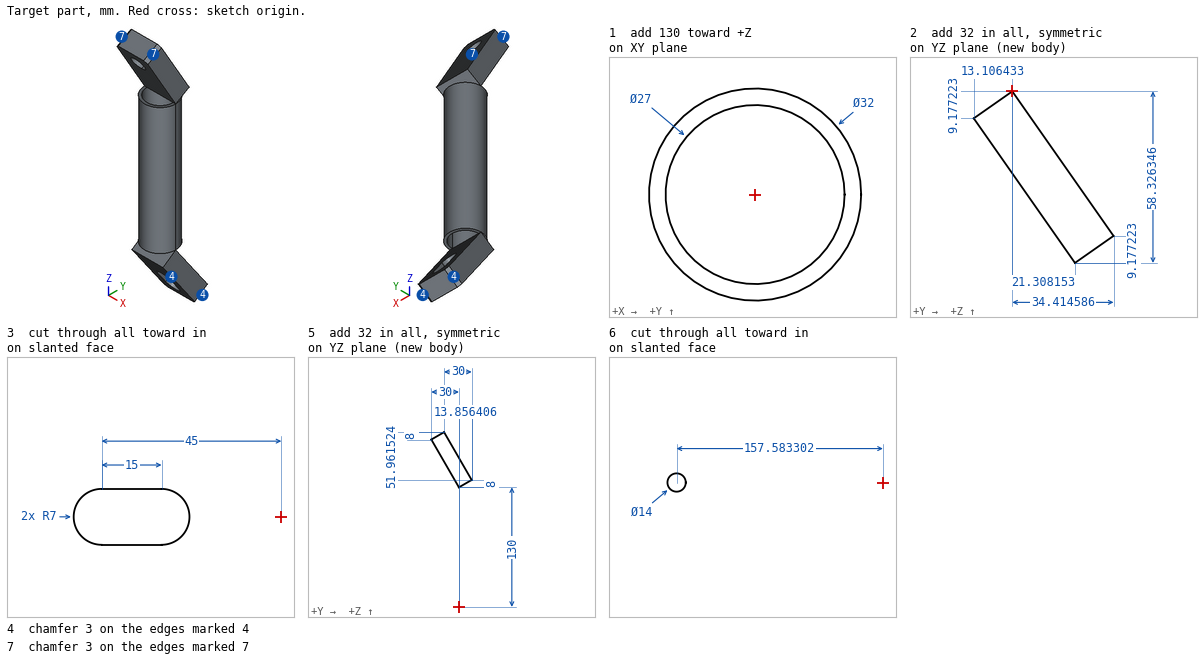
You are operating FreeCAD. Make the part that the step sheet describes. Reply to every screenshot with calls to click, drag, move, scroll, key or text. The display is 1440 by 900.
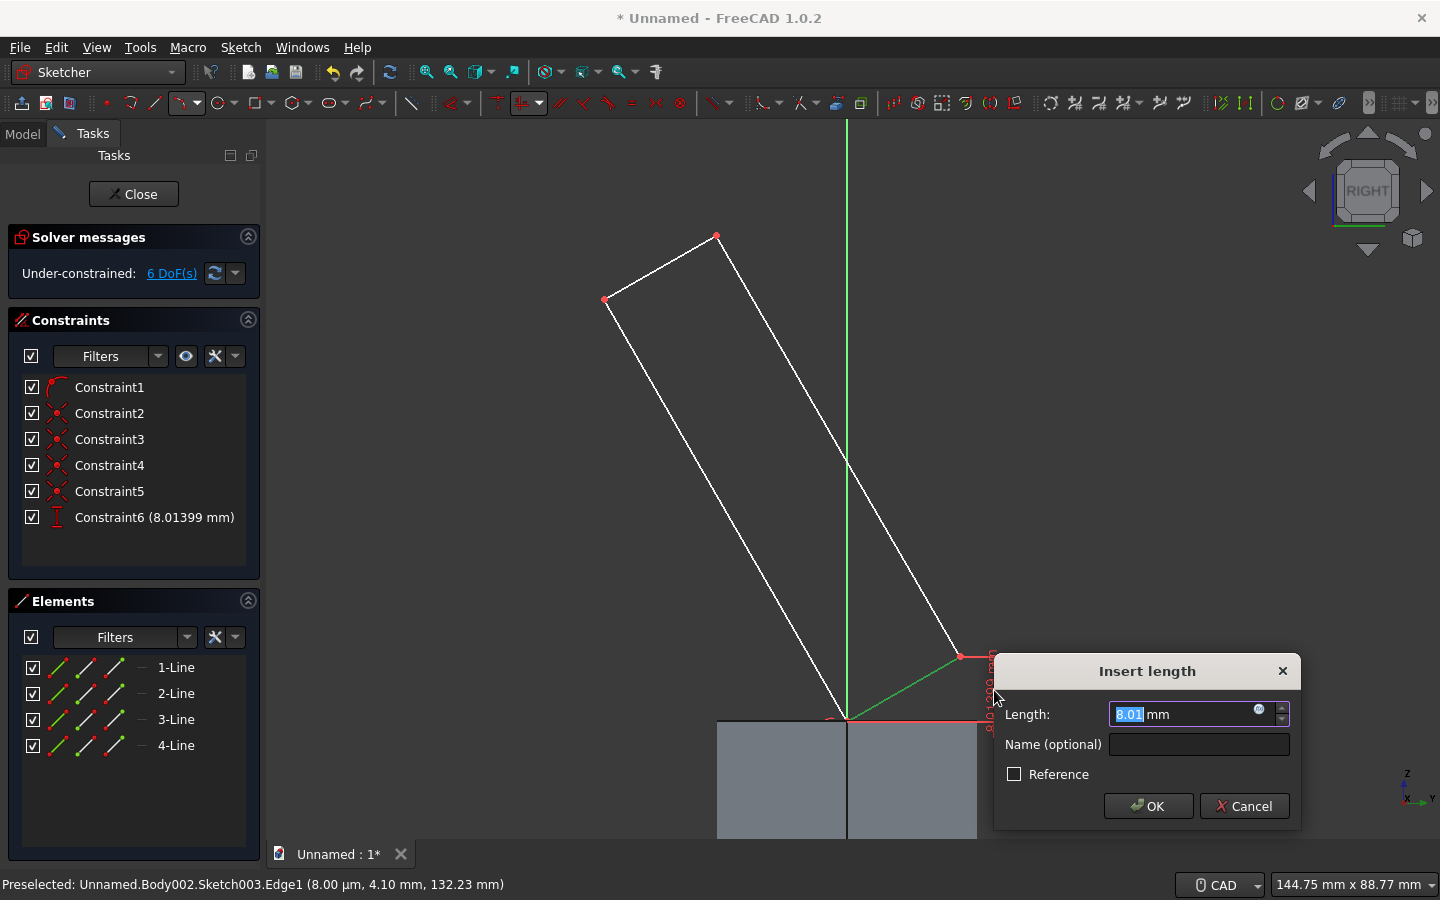
text(8)
key(Return)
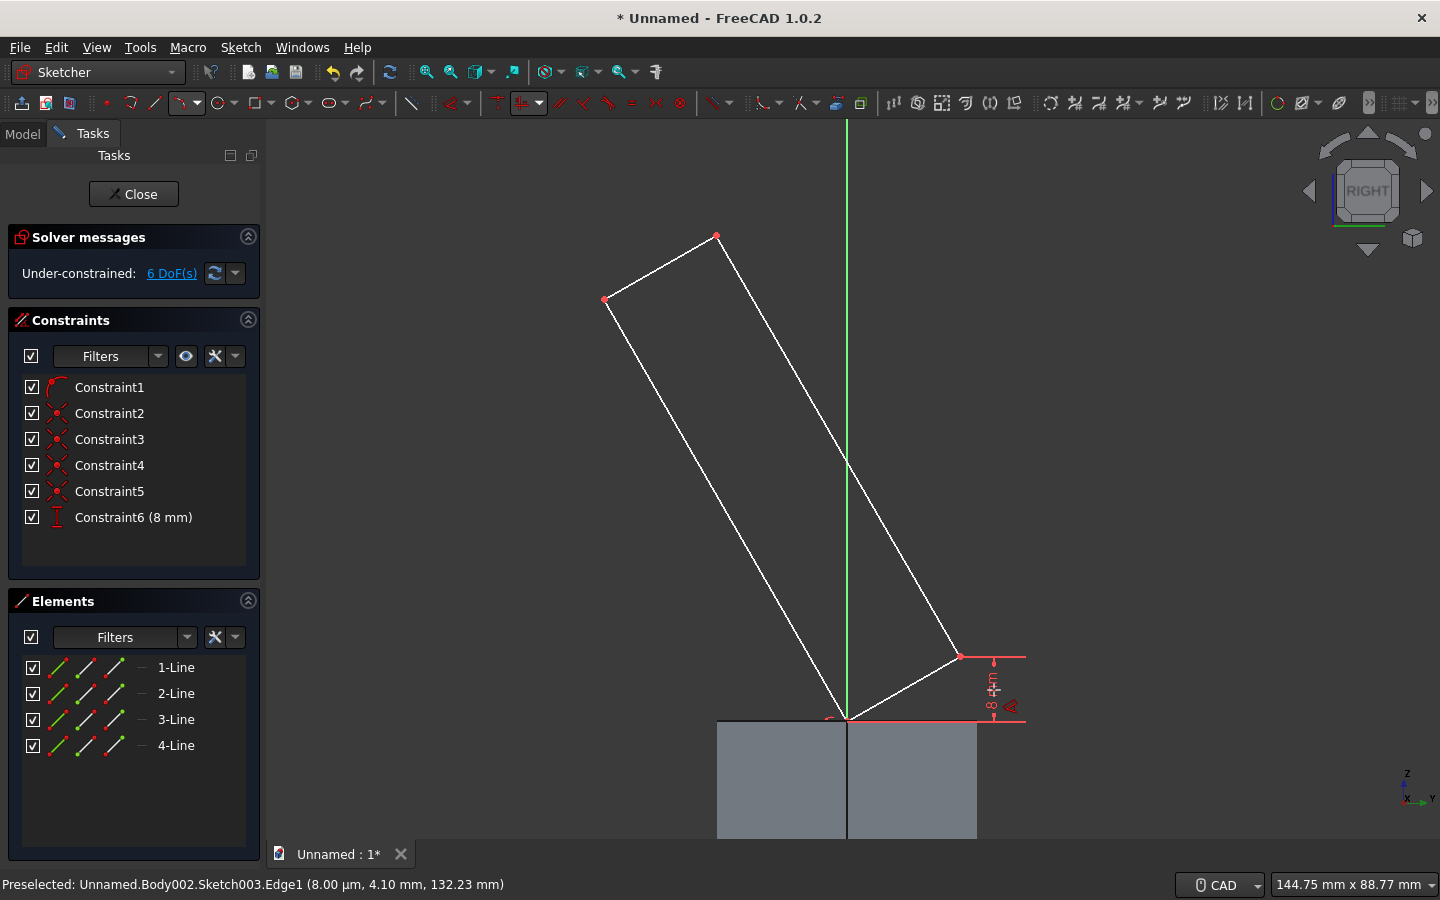
click(682, 255)
click(570, 268)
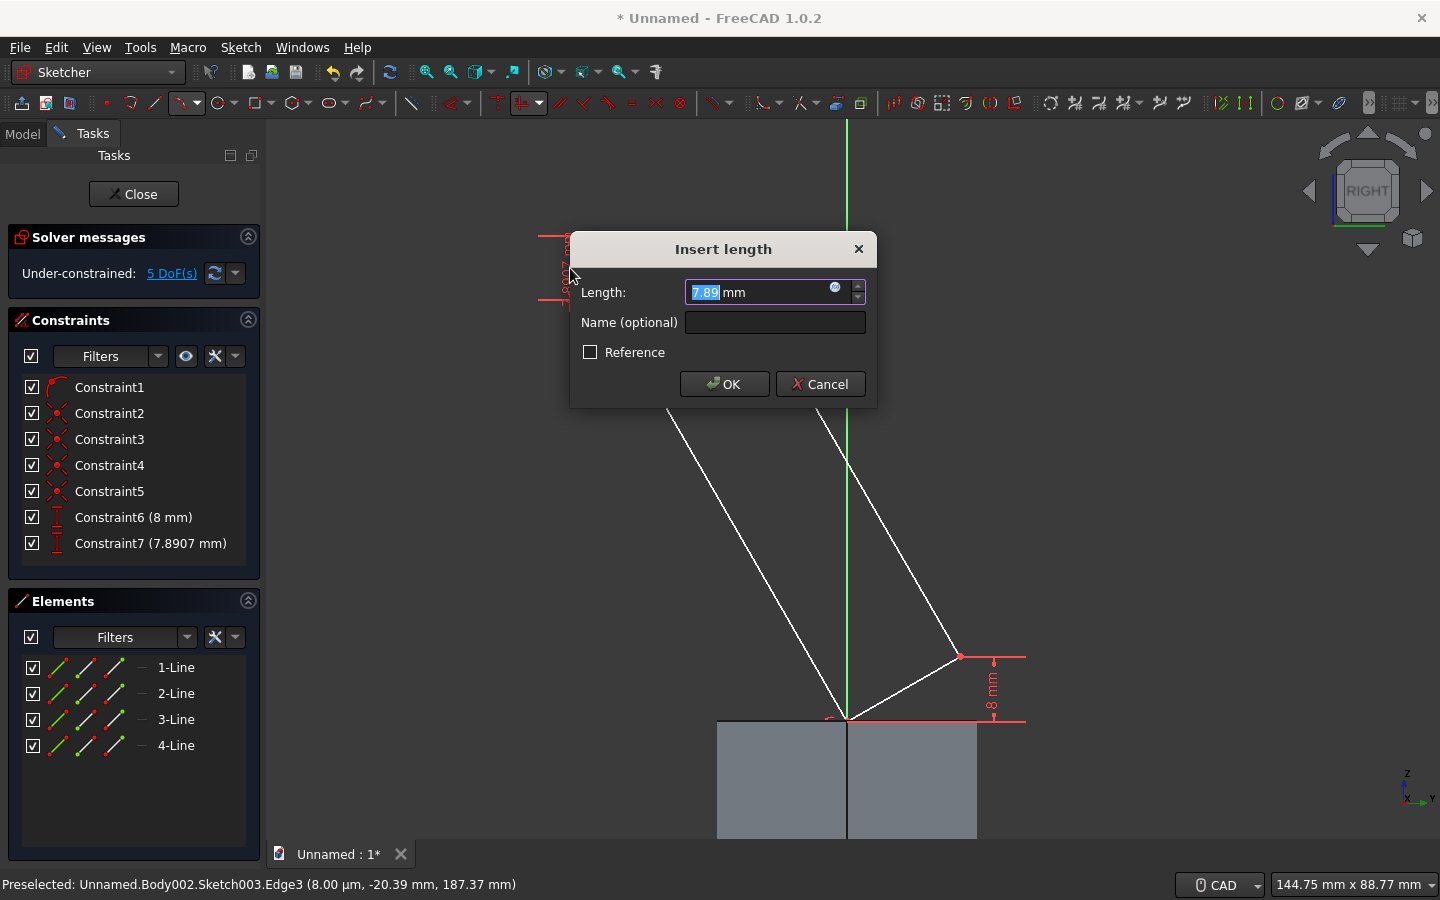
text(8)
key(Return)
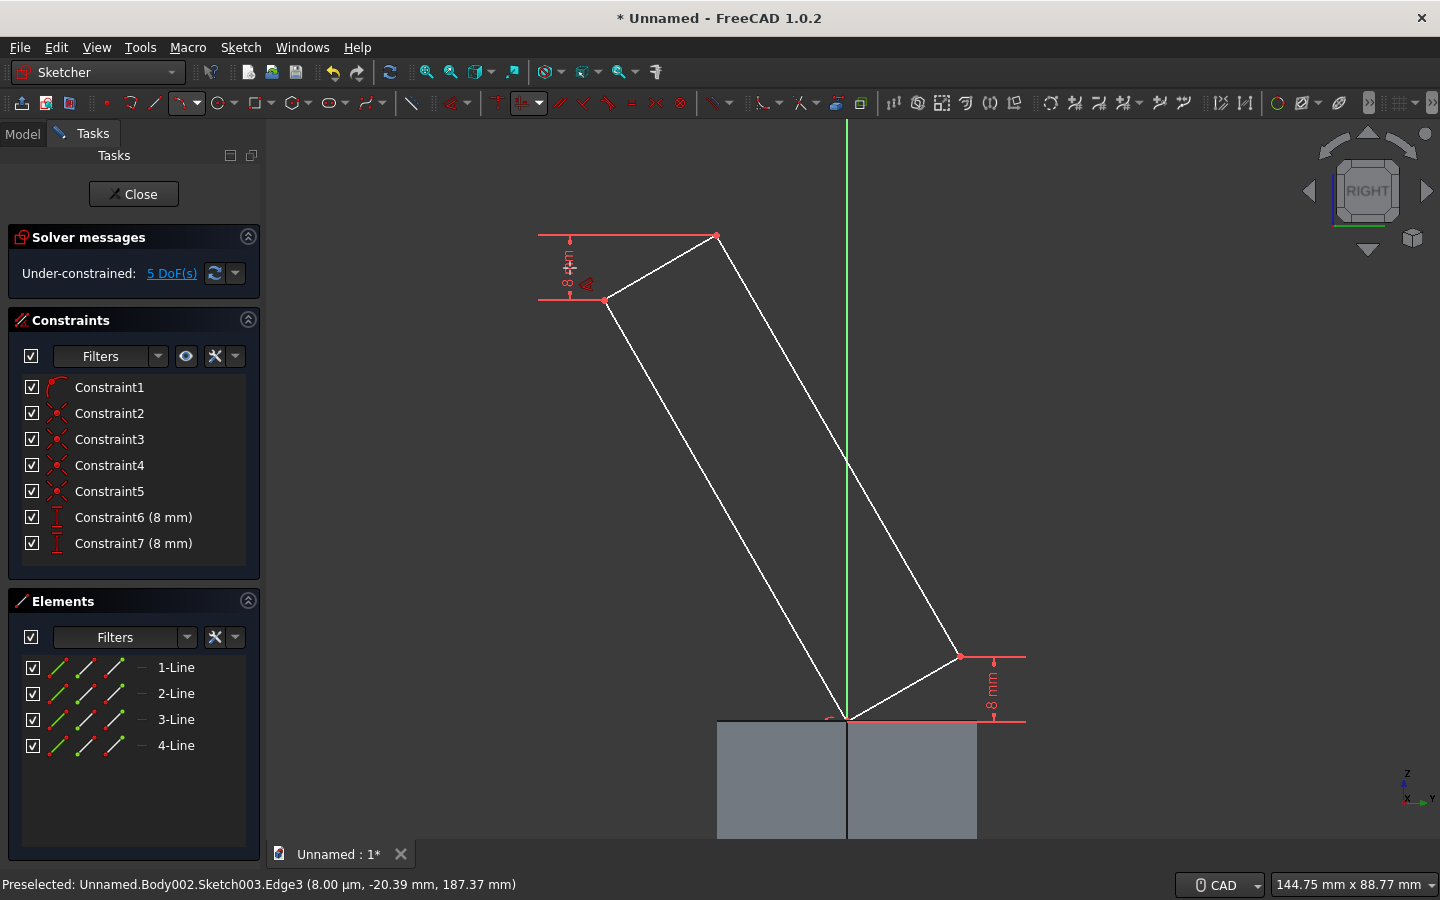
click(604, 300)
click(781, 266)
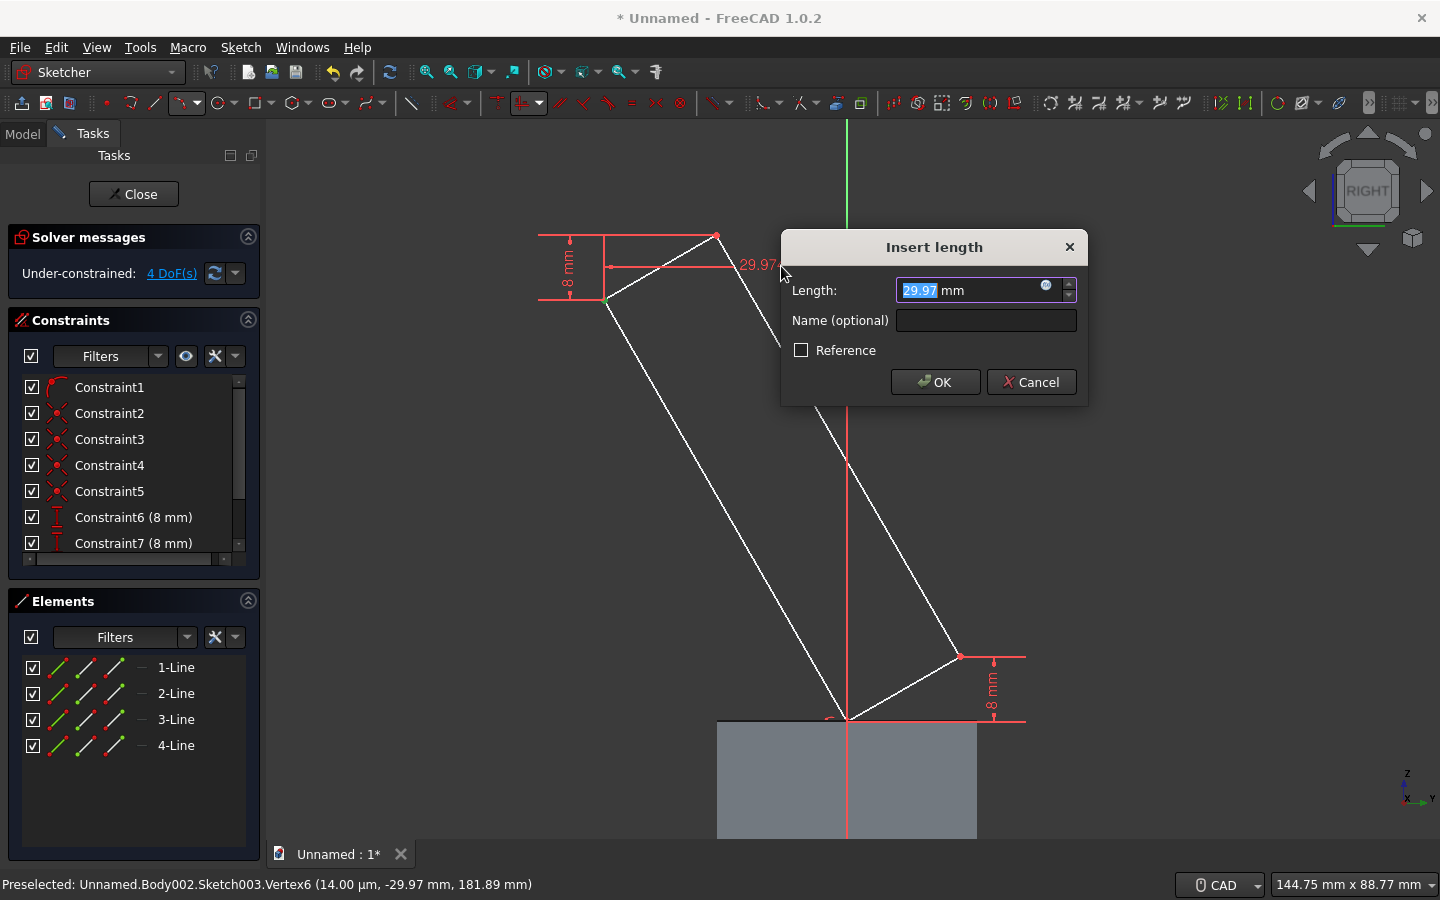
text(30)
key(Return)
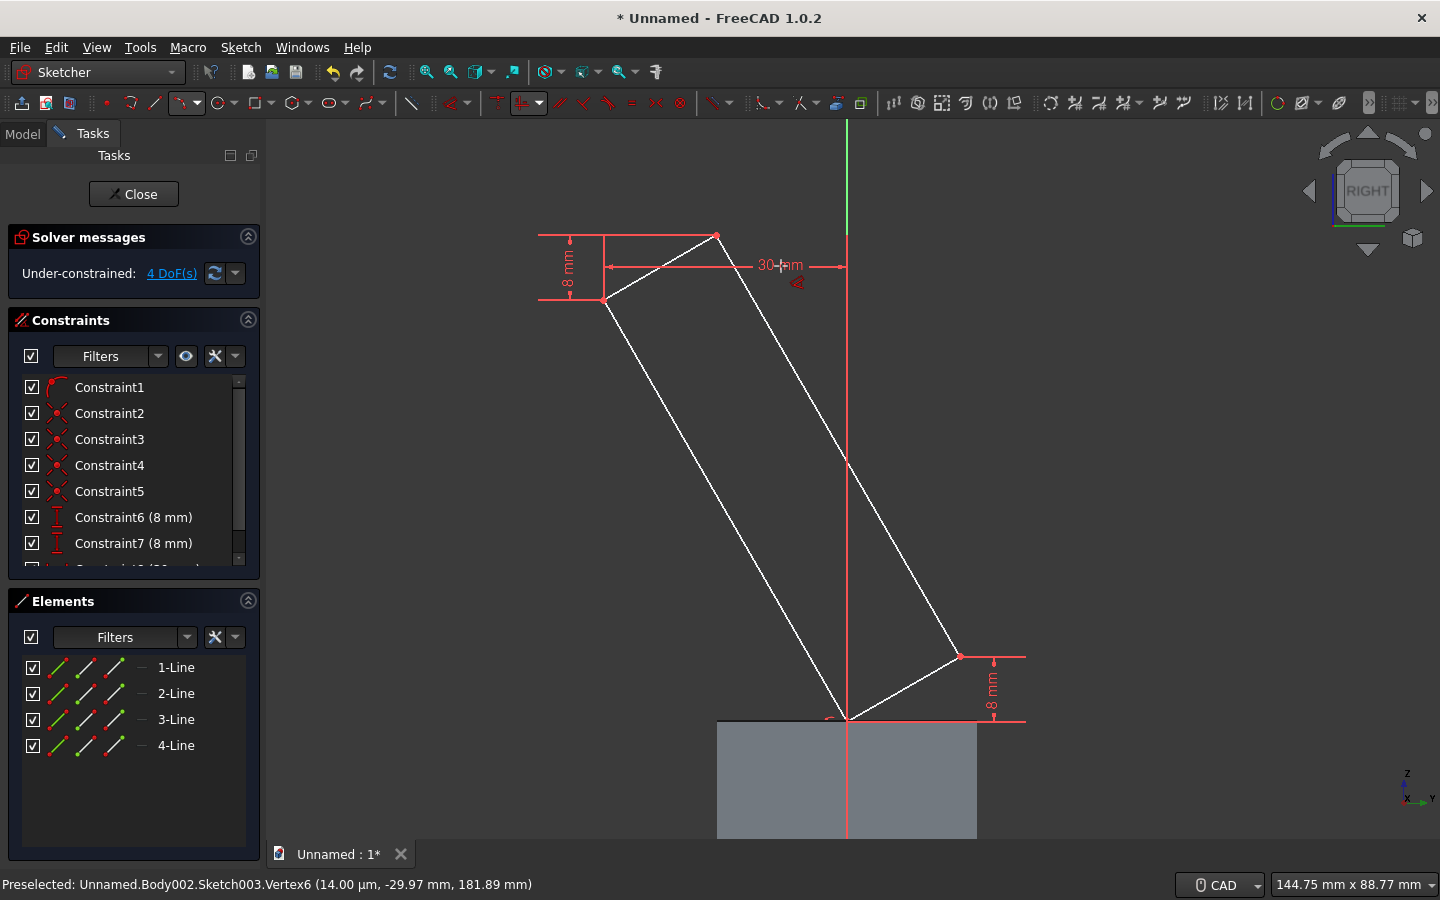
click(887, 530)
click(782, 201)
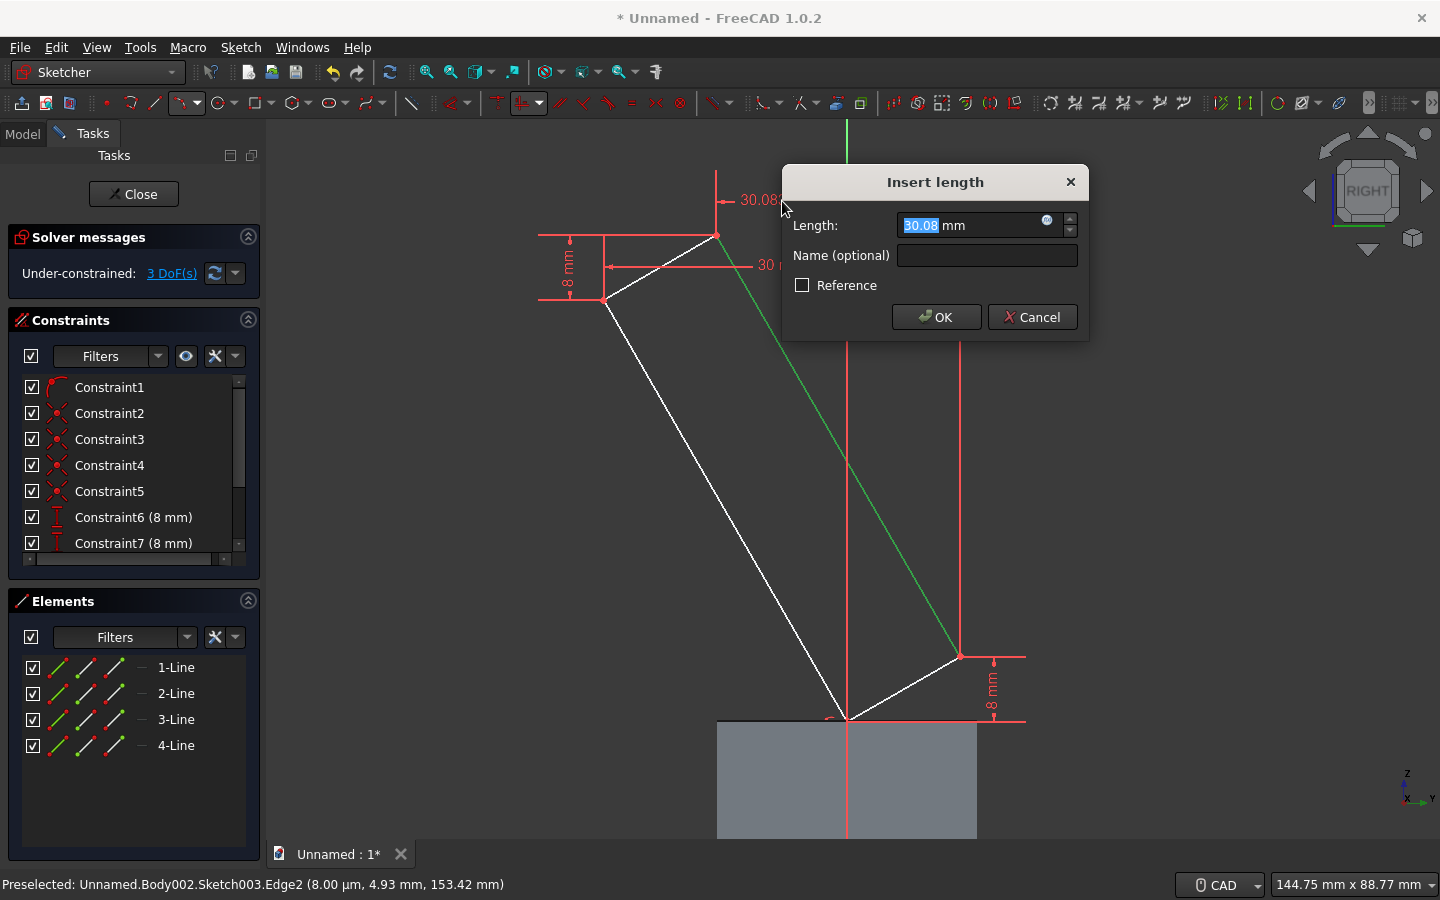
text(30)
key(Return)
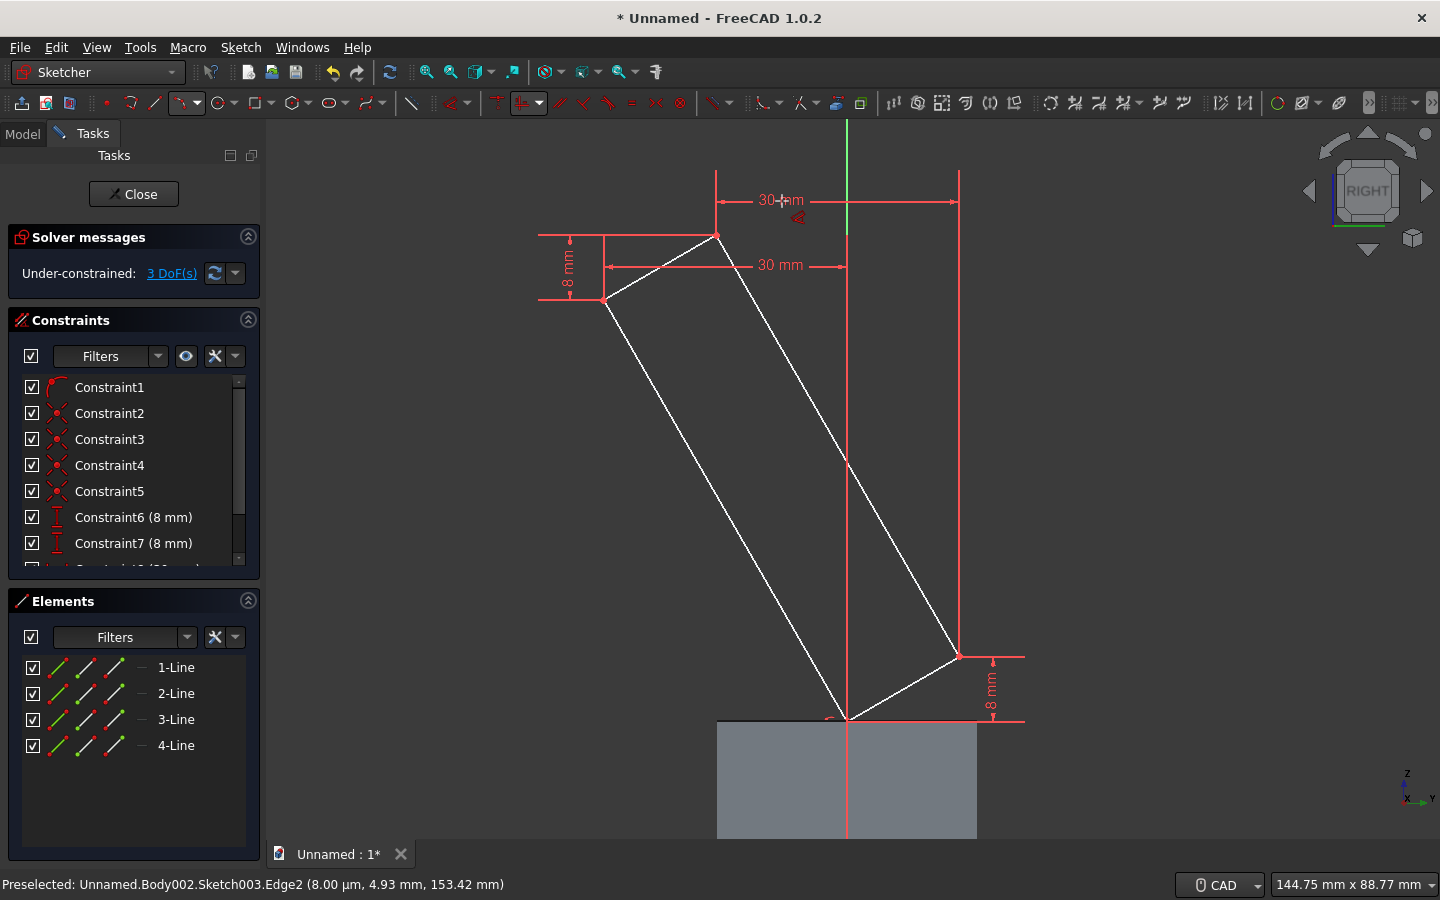
click(847, 722)
click(881, 766)